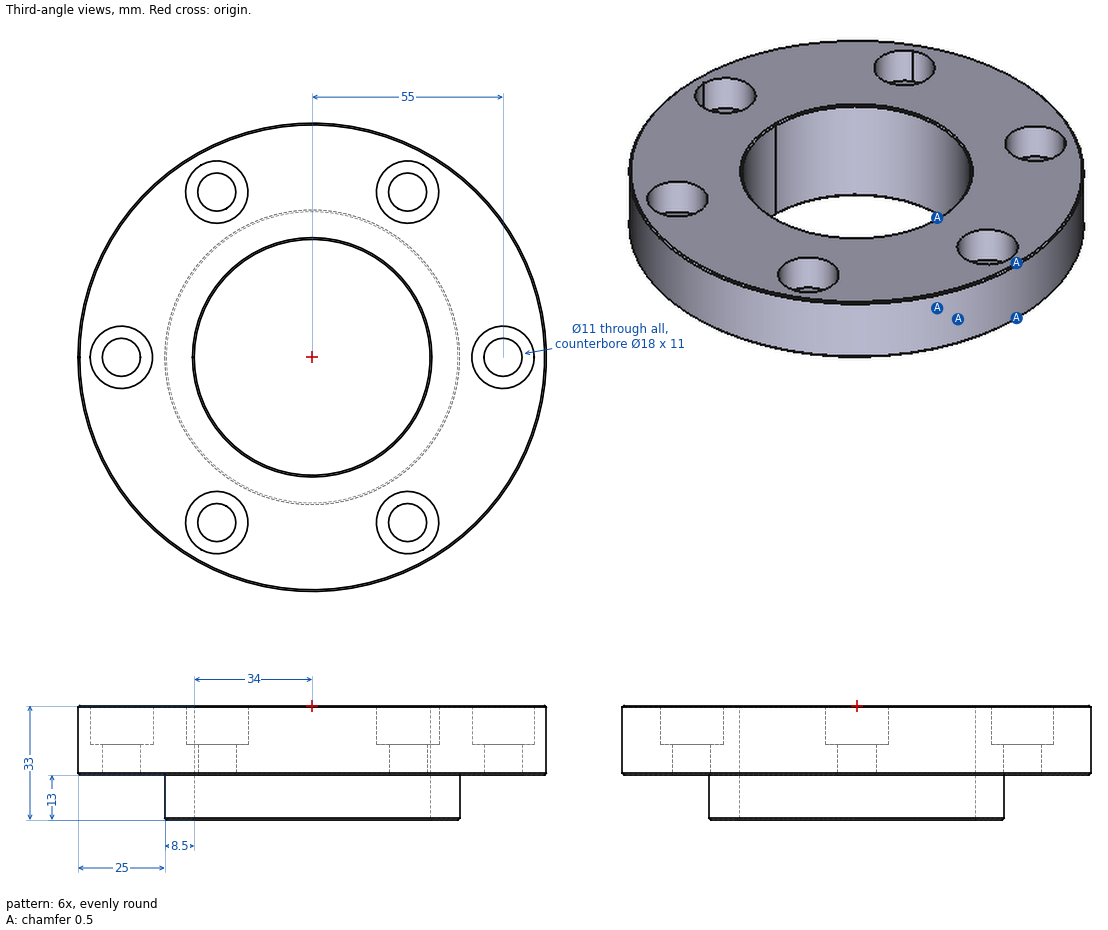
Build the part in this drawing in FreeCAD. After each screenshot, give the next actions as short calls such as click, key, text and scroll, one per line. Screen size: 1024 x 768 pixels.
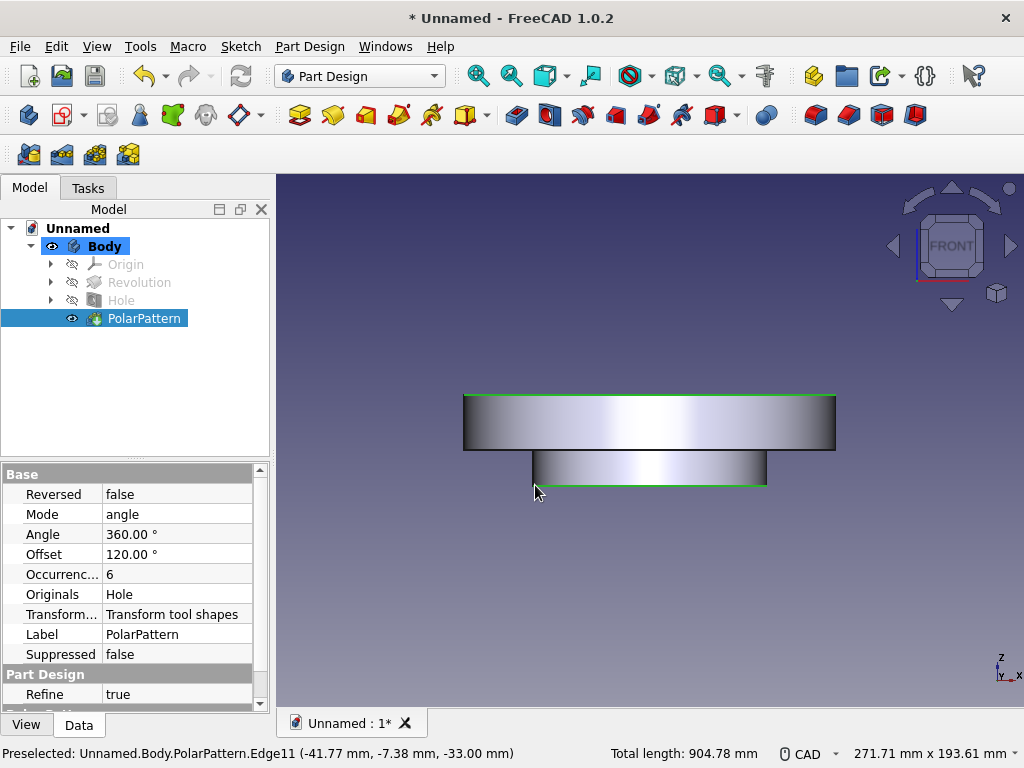
click(800, 449, ctrl)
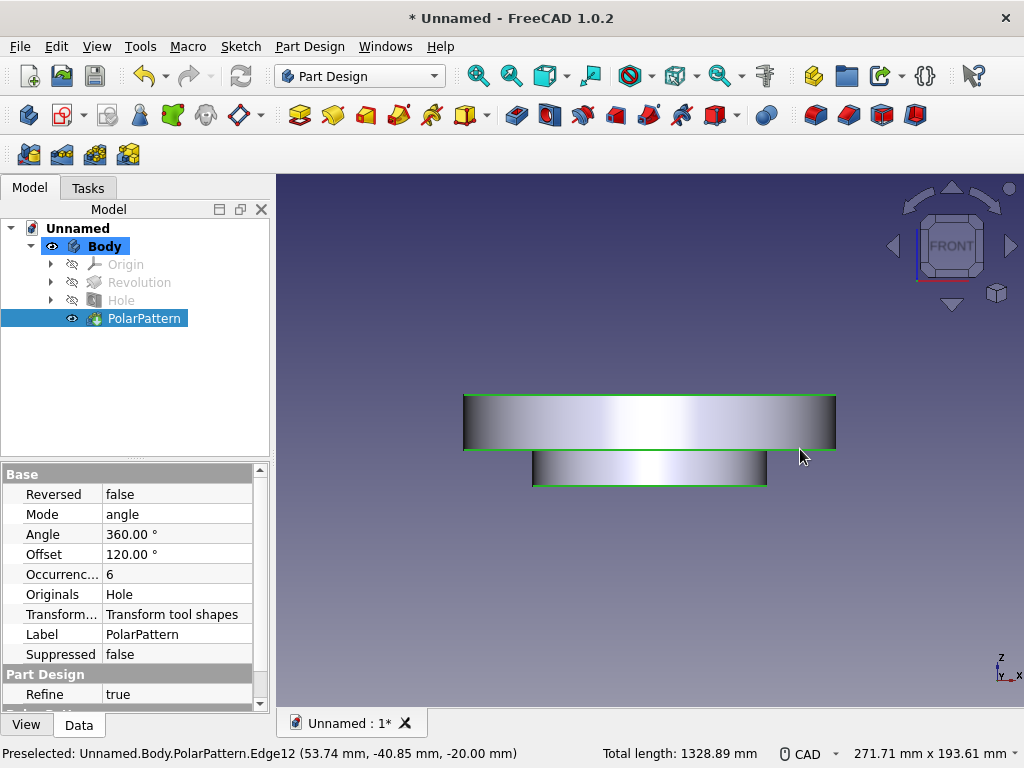
key(3)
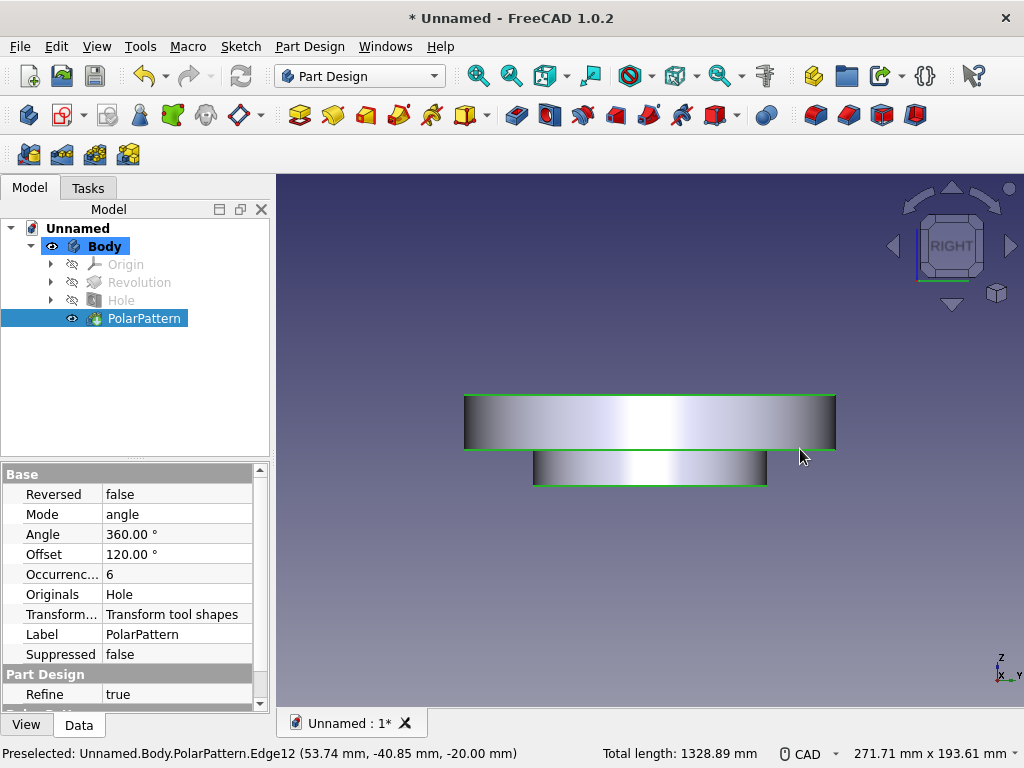
key(5)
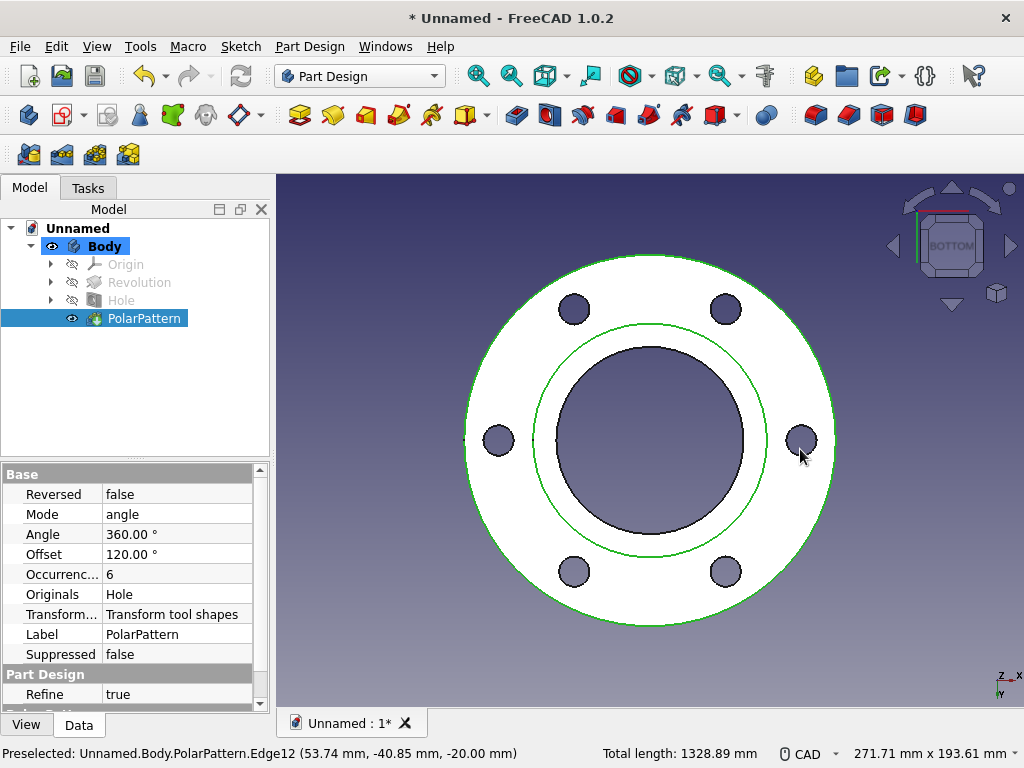
click(744, 440, ctrl)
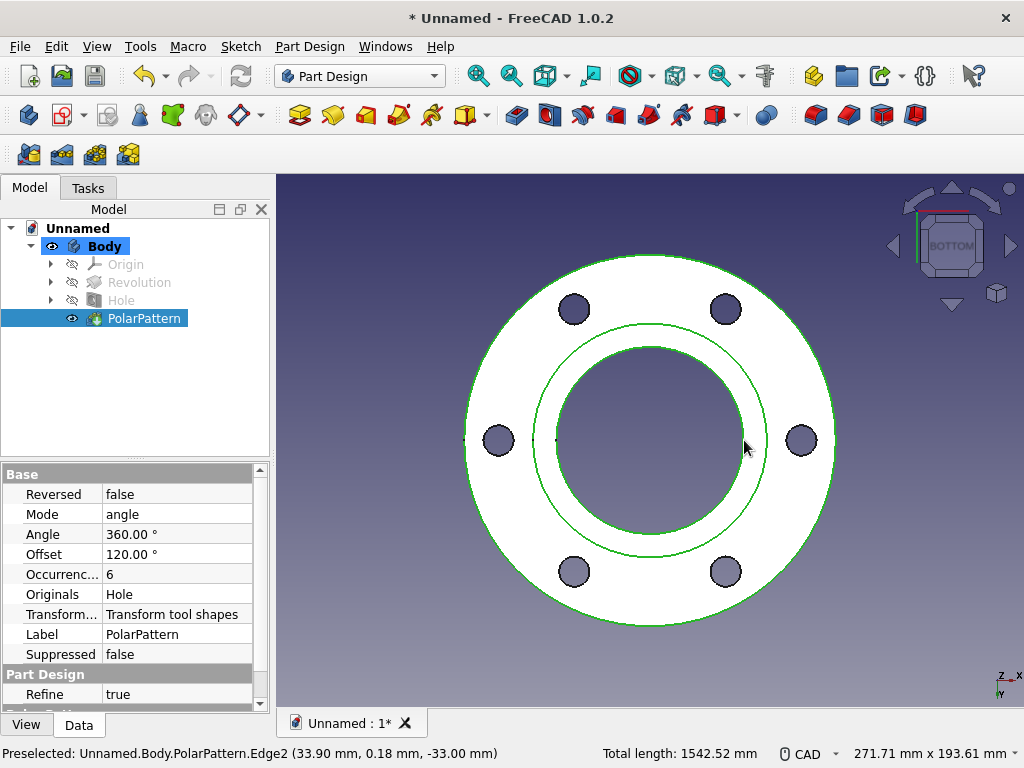
click(849, 116)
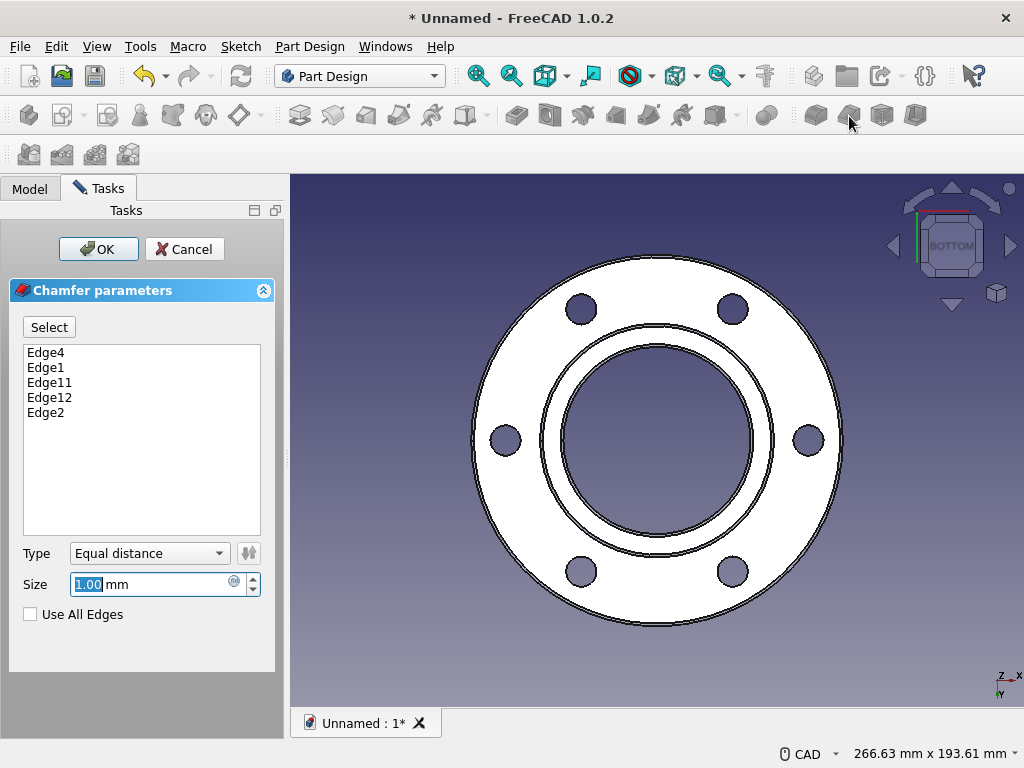
text(0.5)
key(Tab)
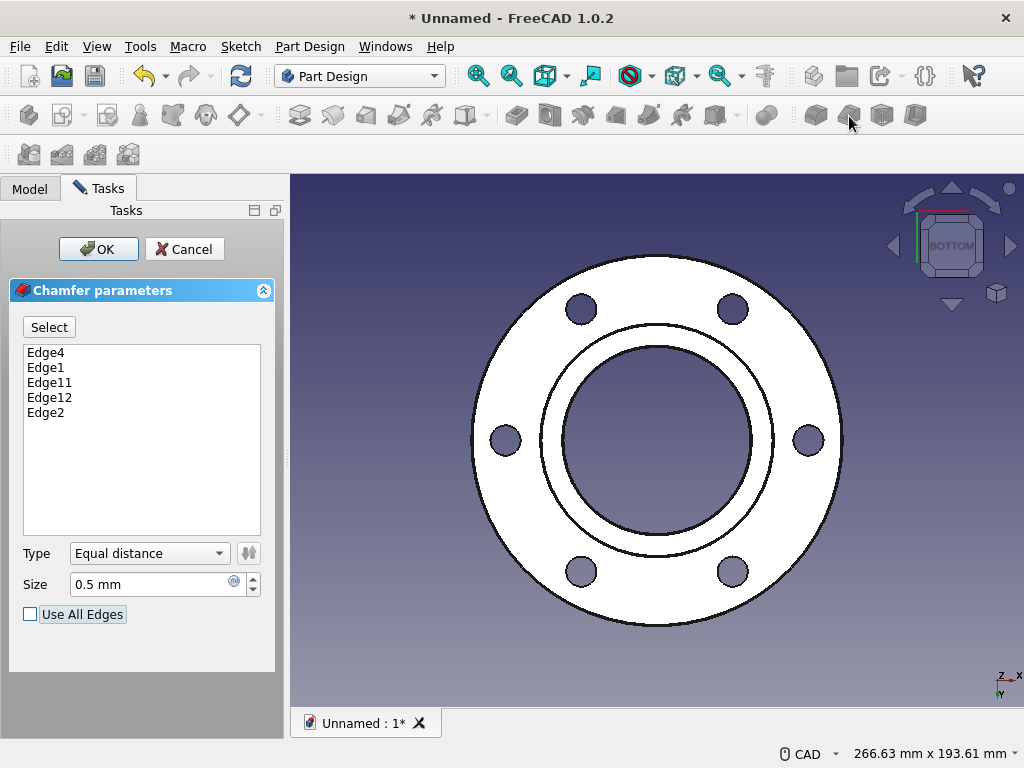
click(99, 249)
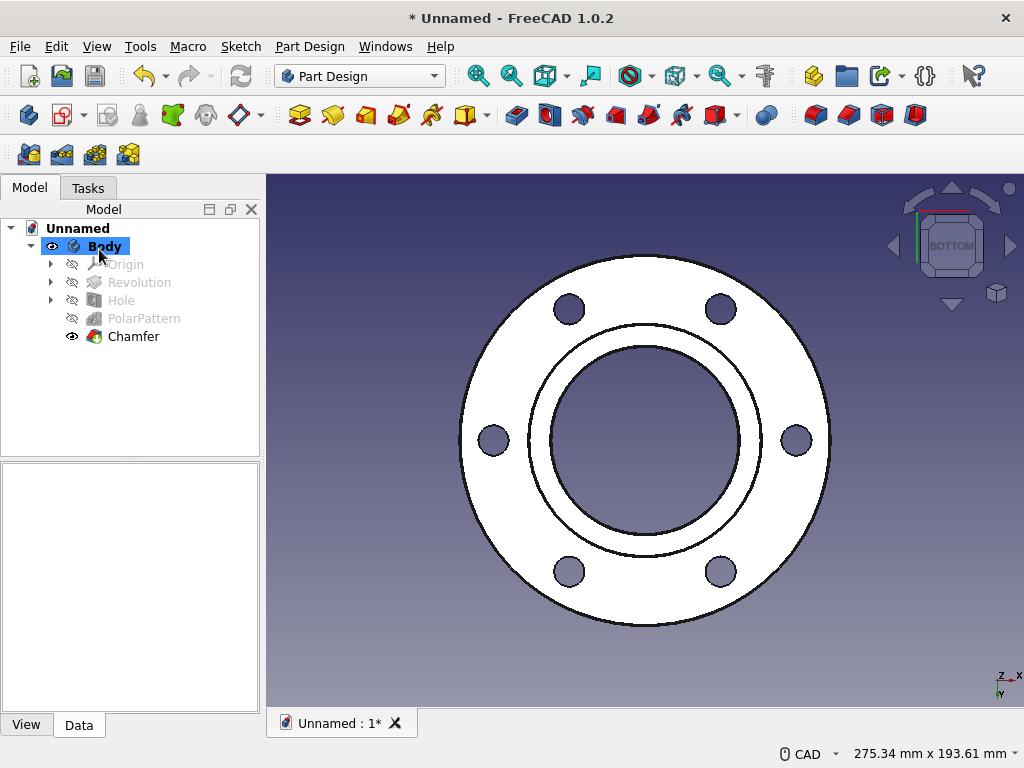
key(0)